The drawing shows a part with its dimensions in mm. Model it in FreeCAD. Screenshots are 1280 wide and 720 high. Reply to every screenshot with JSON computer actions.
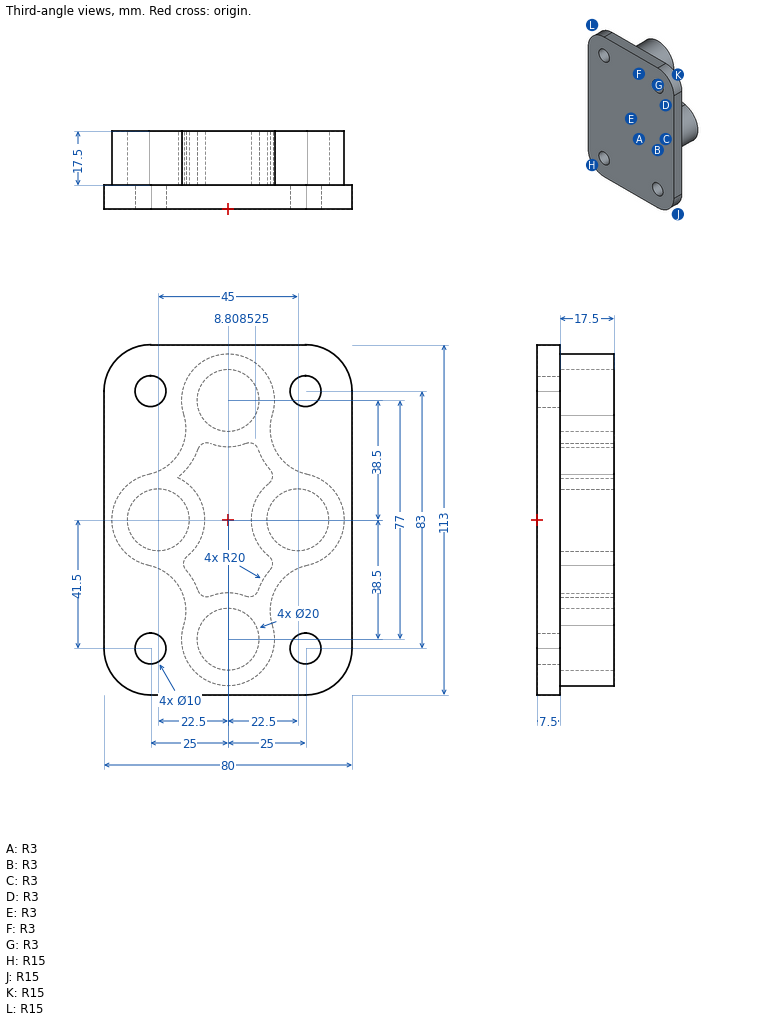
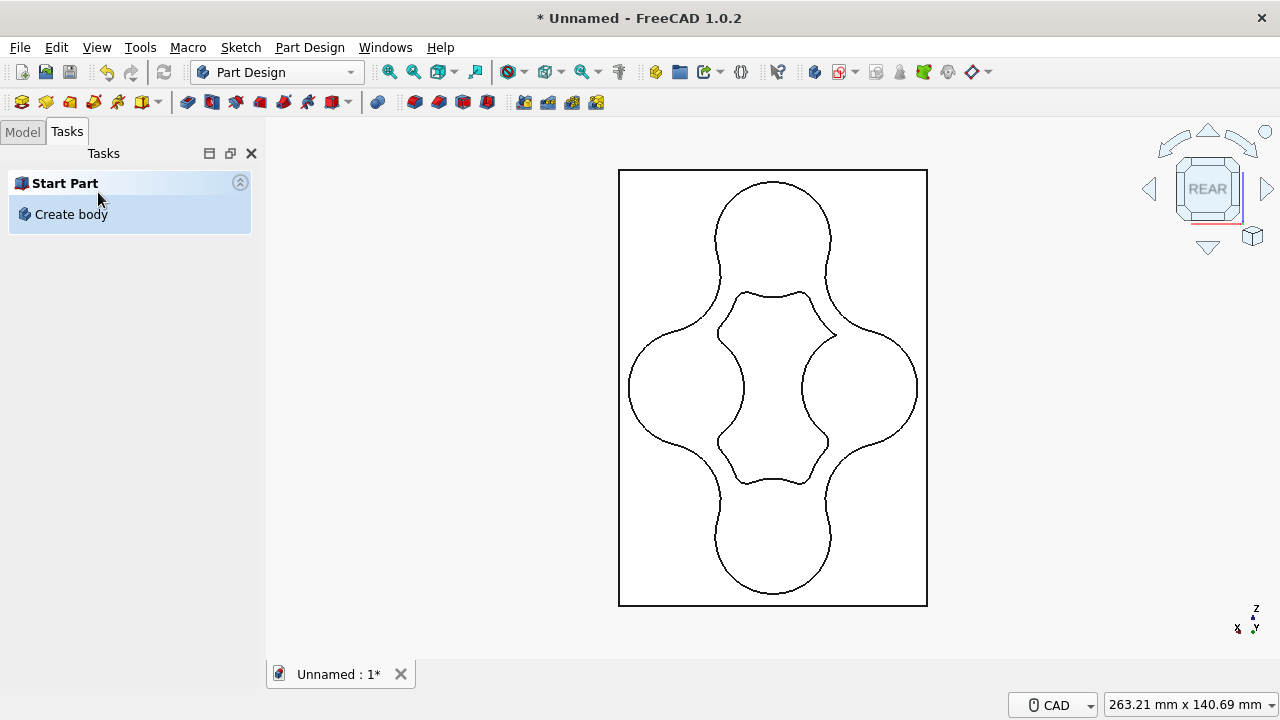
{"action": "left_click", "coordinate": [690, 387]}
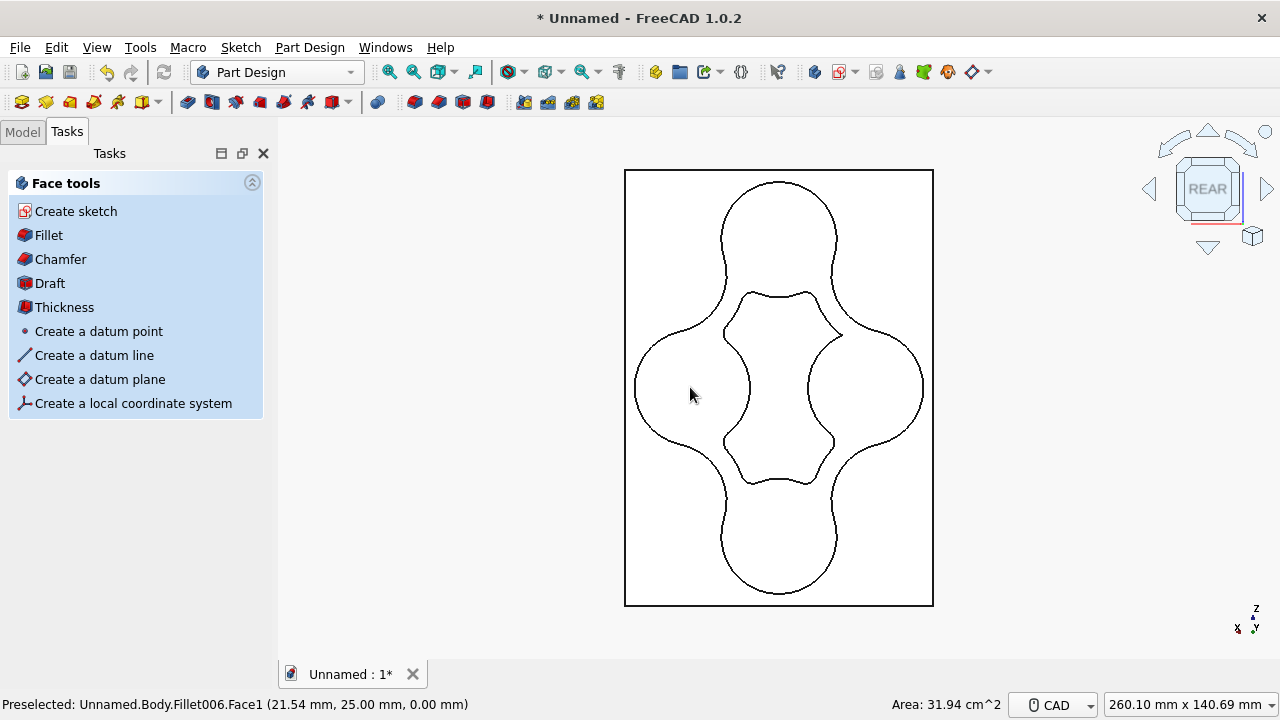
{"action": "left_click", "coordinate": [840, 72]}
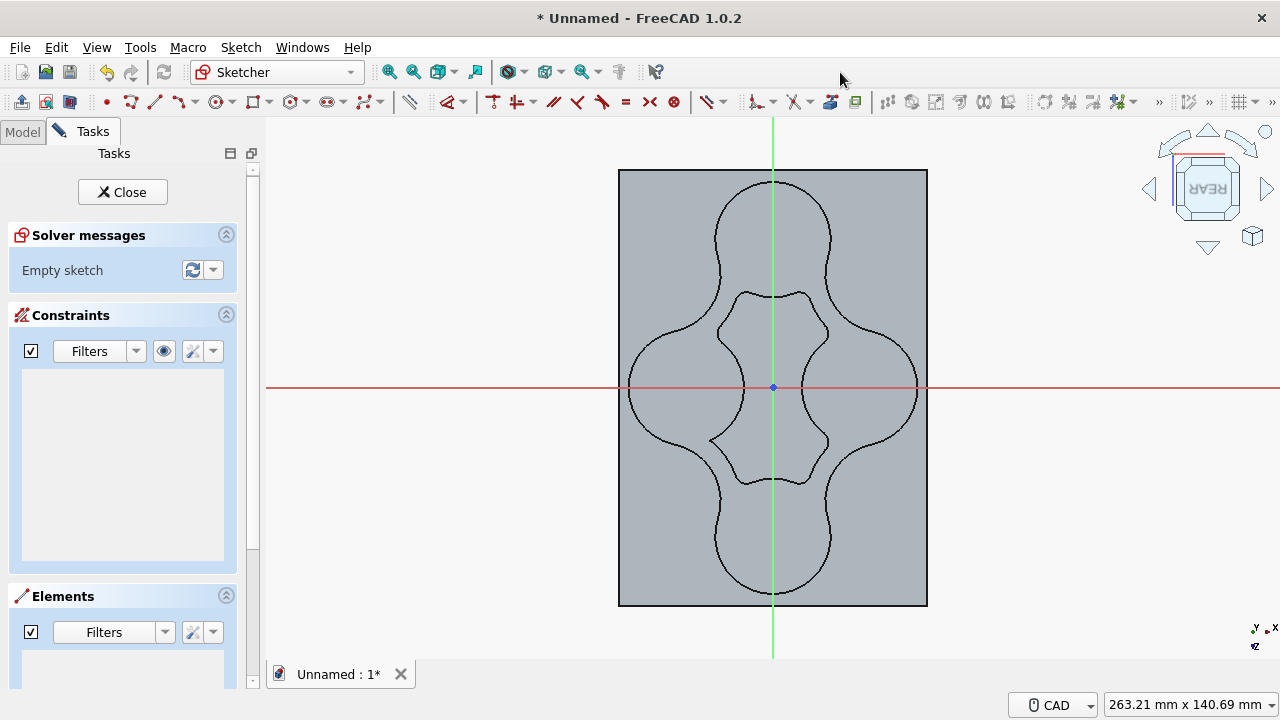
{"action": "key", "text": "g c"}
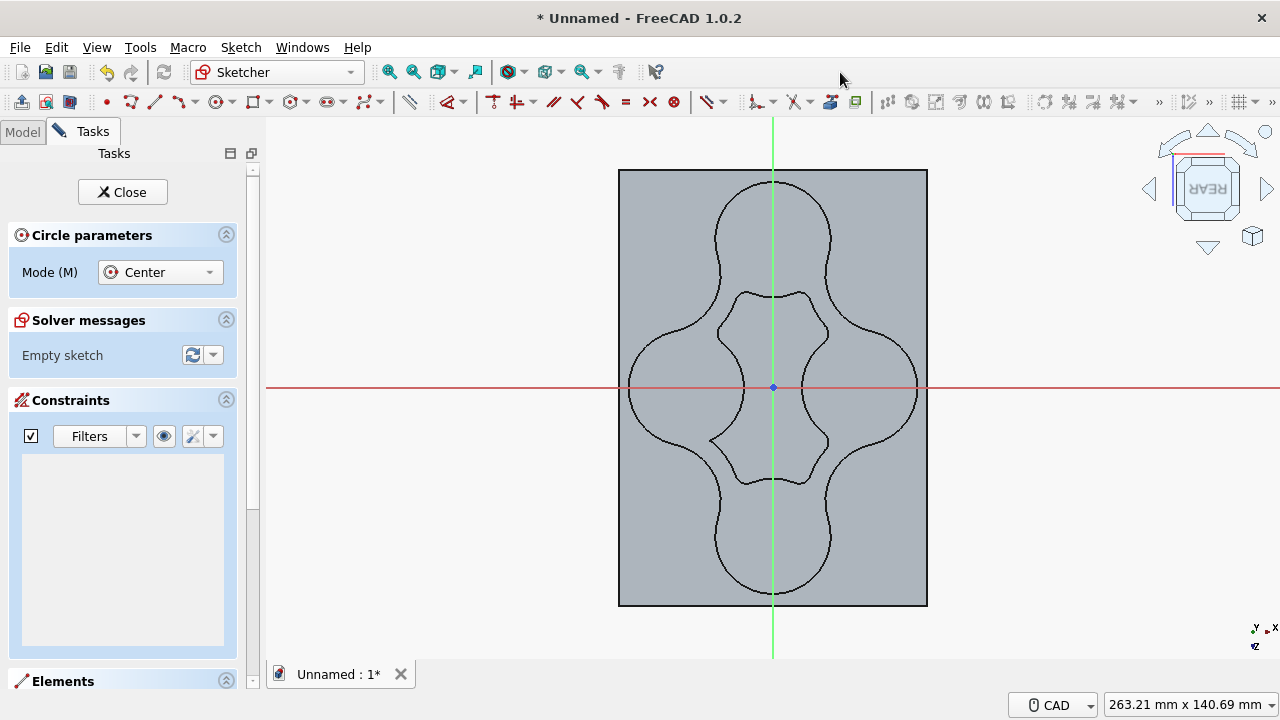
{"action": "left_click", "coordinate": [773, 240]}
{"action": "mouse_move", "coordinate": [800, 212]}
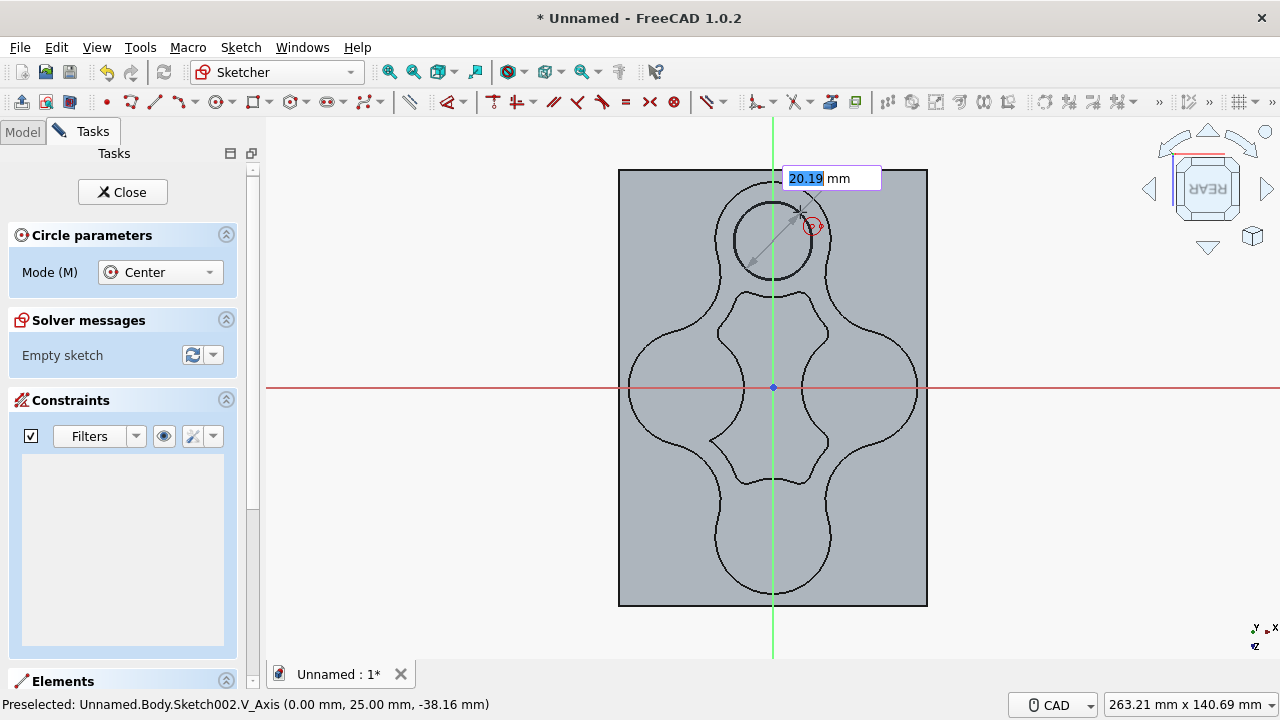
{"action": "type", "text": "20"}
{"action": "key", "text": "Return"}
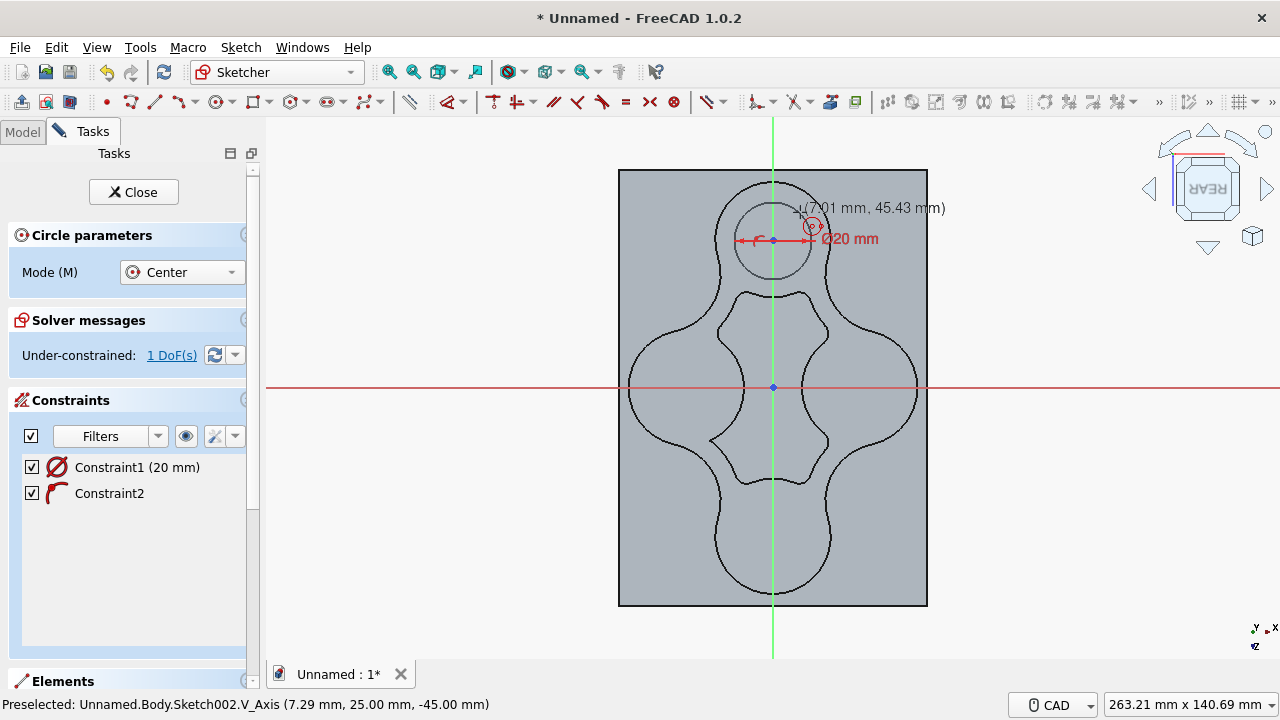
{"action": "left_click", "coordinate": [860, 388]}
{"action": "mouse_move", "coordinate": [887, 361]}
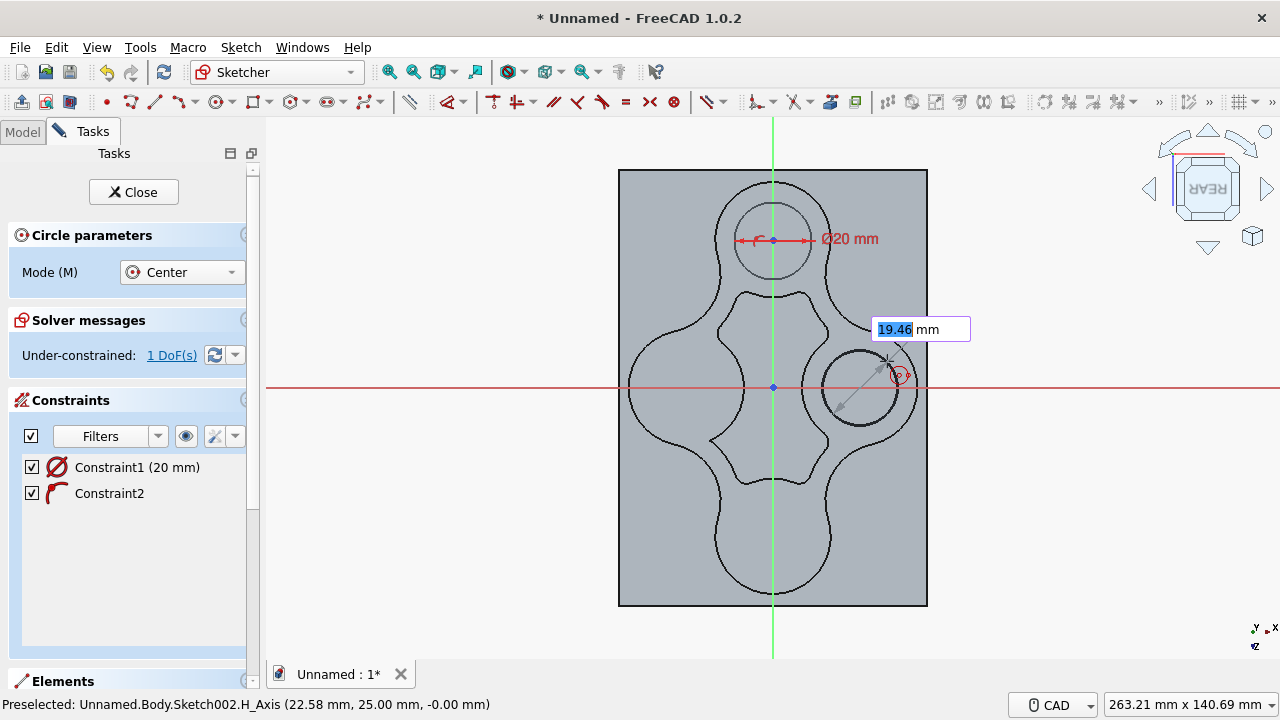
{"action": "type", "text": "20"}
{"action": "key", "text": "Return"}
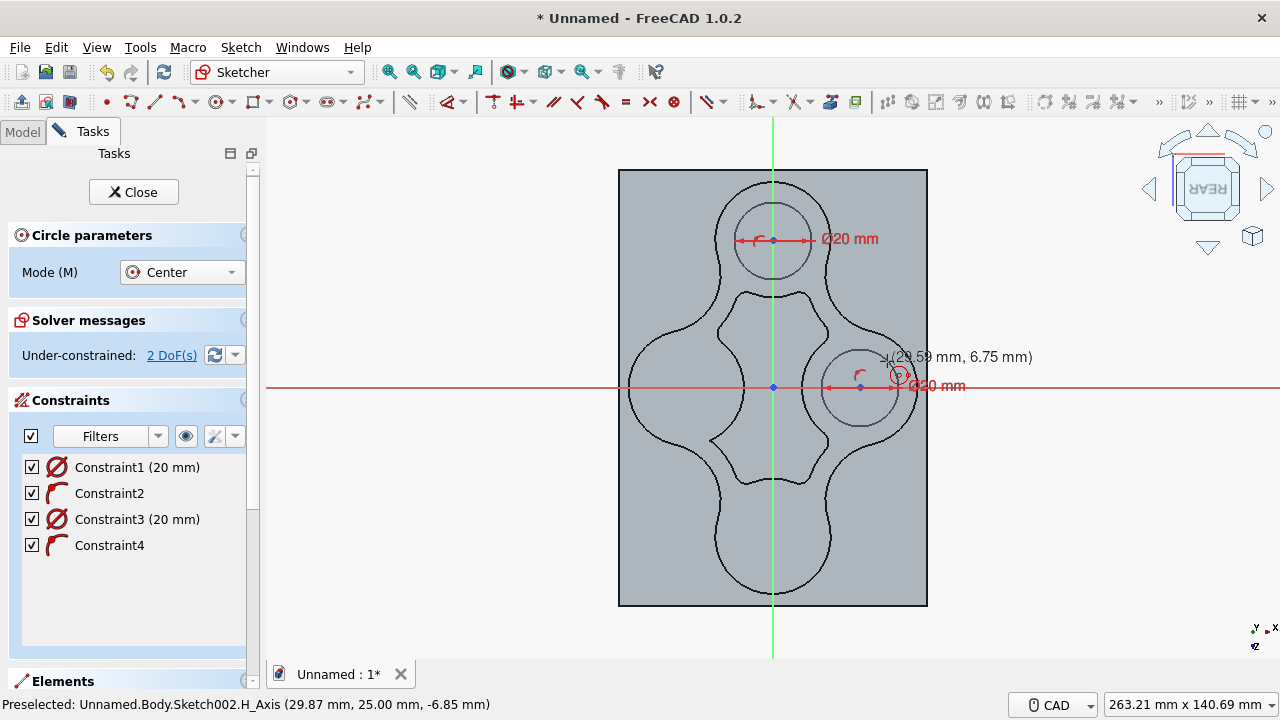
{"action": "left_click", "coordinate": [773, 536]}
{"action": "mouse_move", "coordinate": [800, 509]}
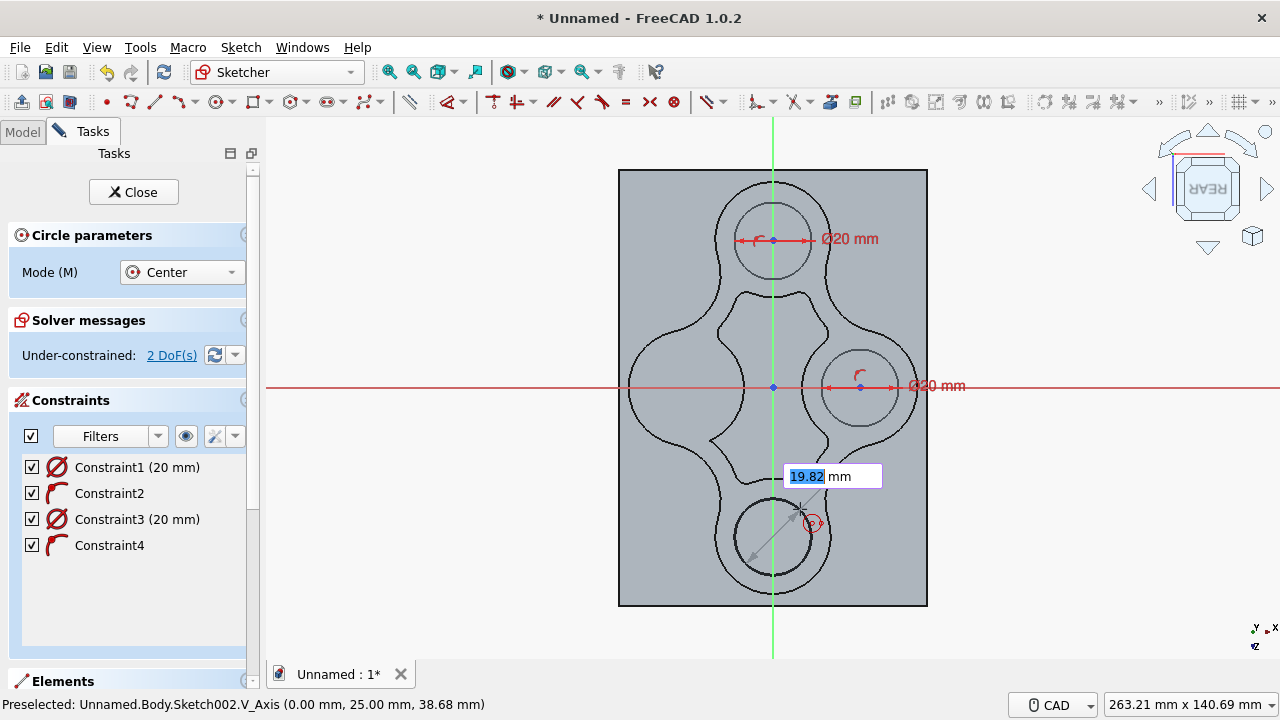
{"action": "type", "text": "20"}
{"action": "key", "text": "Return"}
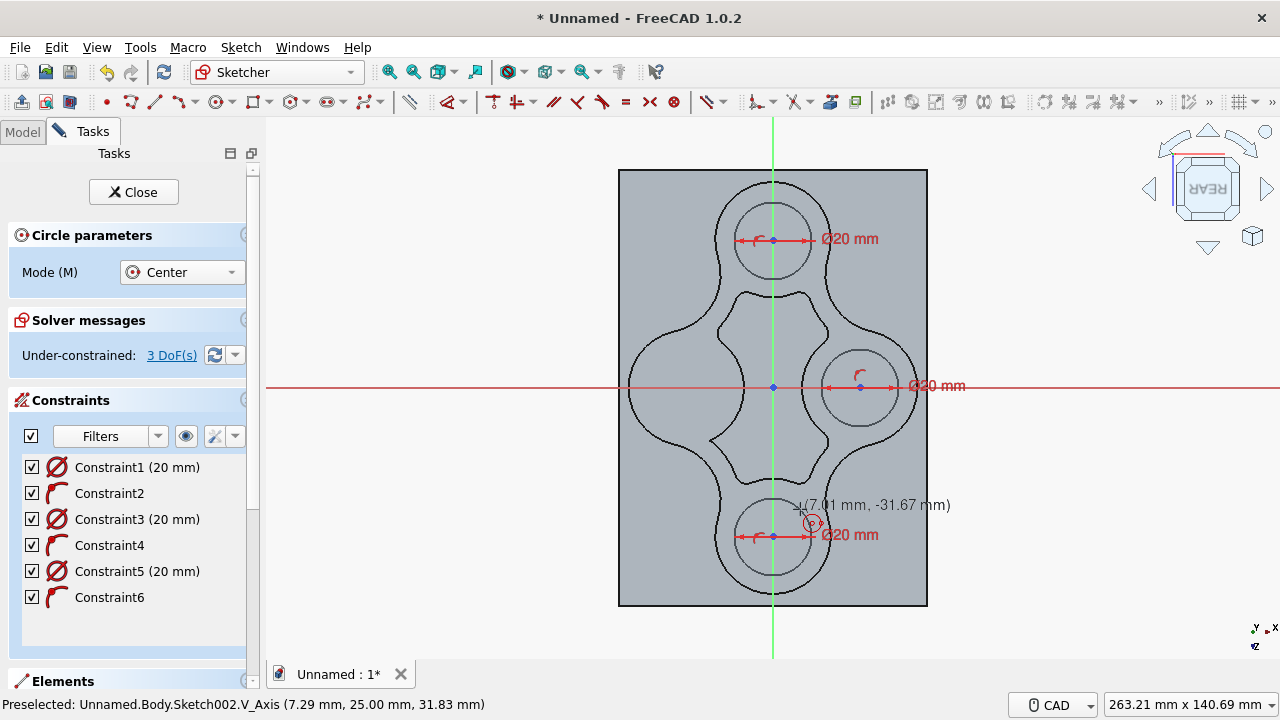
{"action": "left_click", "coordinate": [686, 388]}
{"action": "mouse_move", "coordinate": [714, 361]}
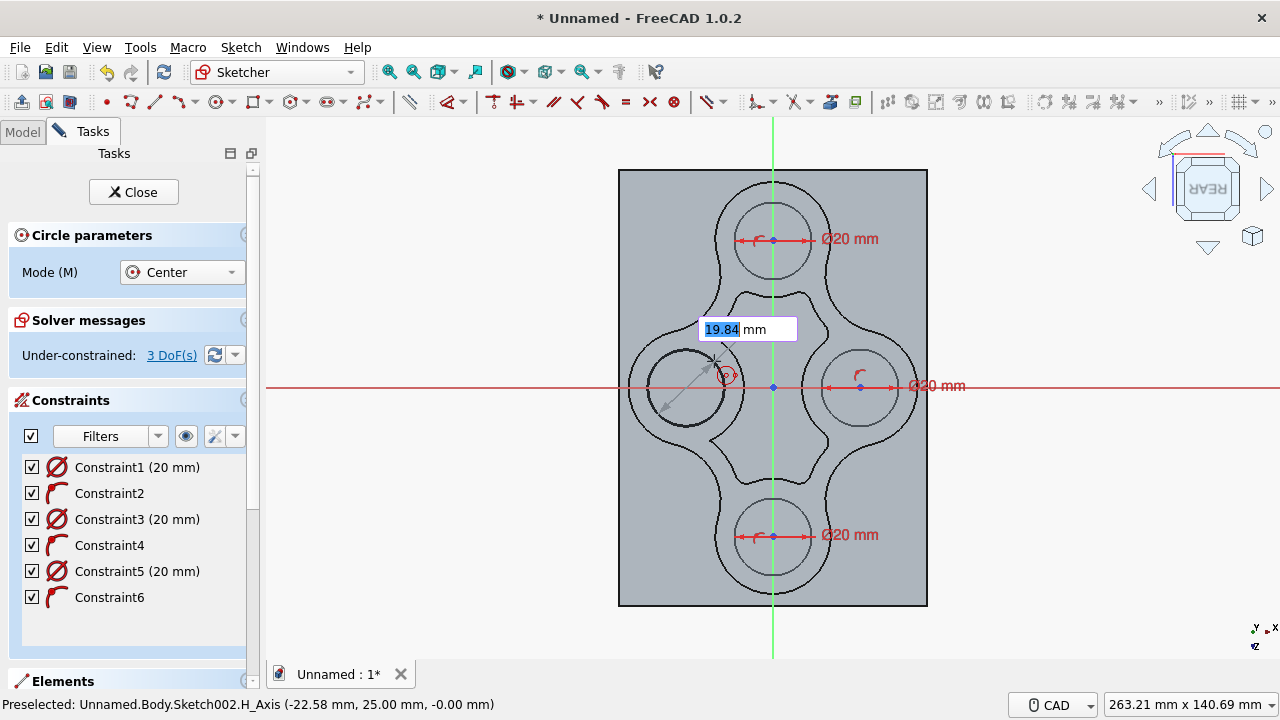
{"action": "type", "text": "20"}
{"action": "key", "text": "Return"}
{"action": "key", "text": "Escape"}